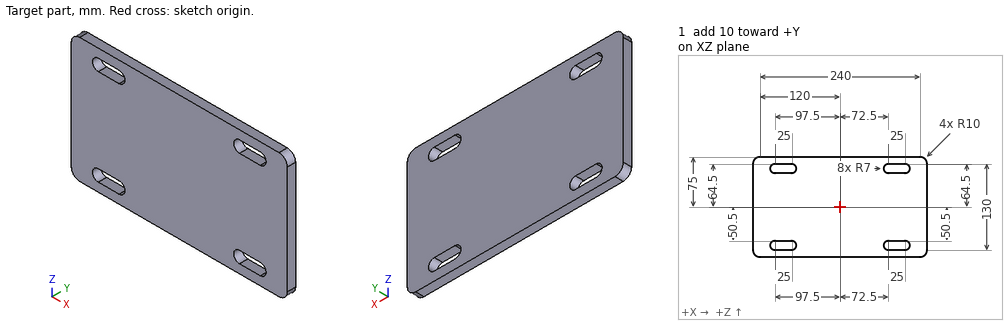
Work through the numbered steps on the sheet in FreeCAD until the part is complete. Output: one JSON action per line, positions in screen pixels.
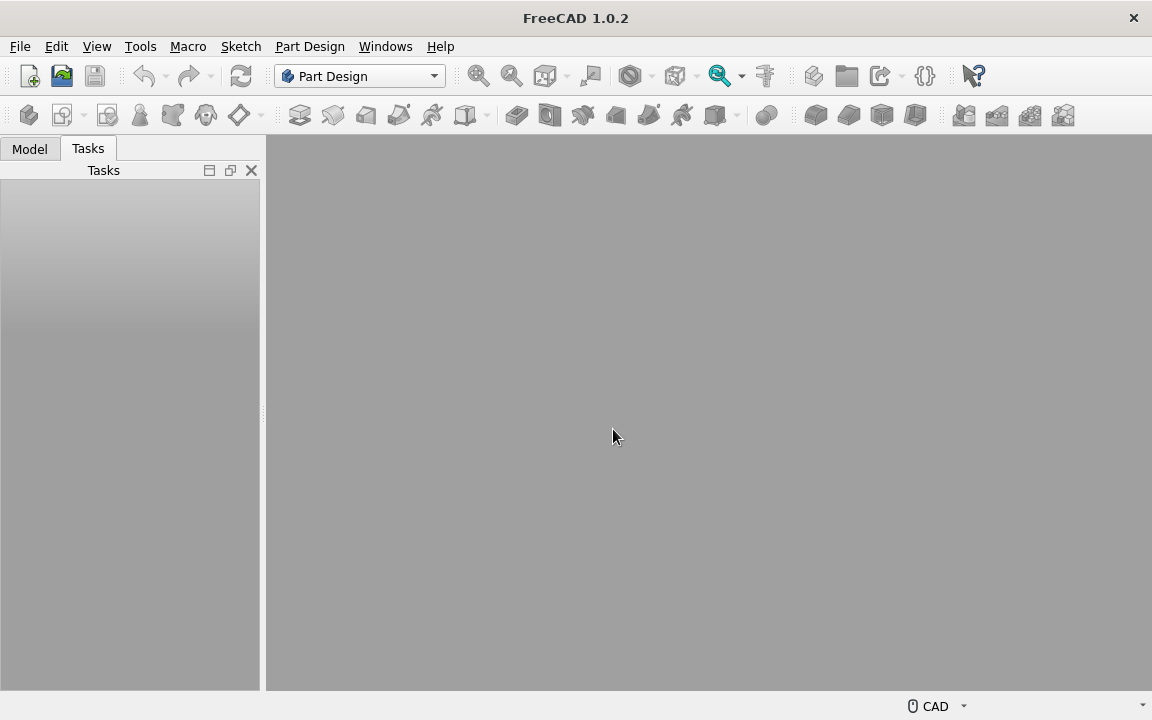
{"action": "left_click", "coordinate": [29, 76]}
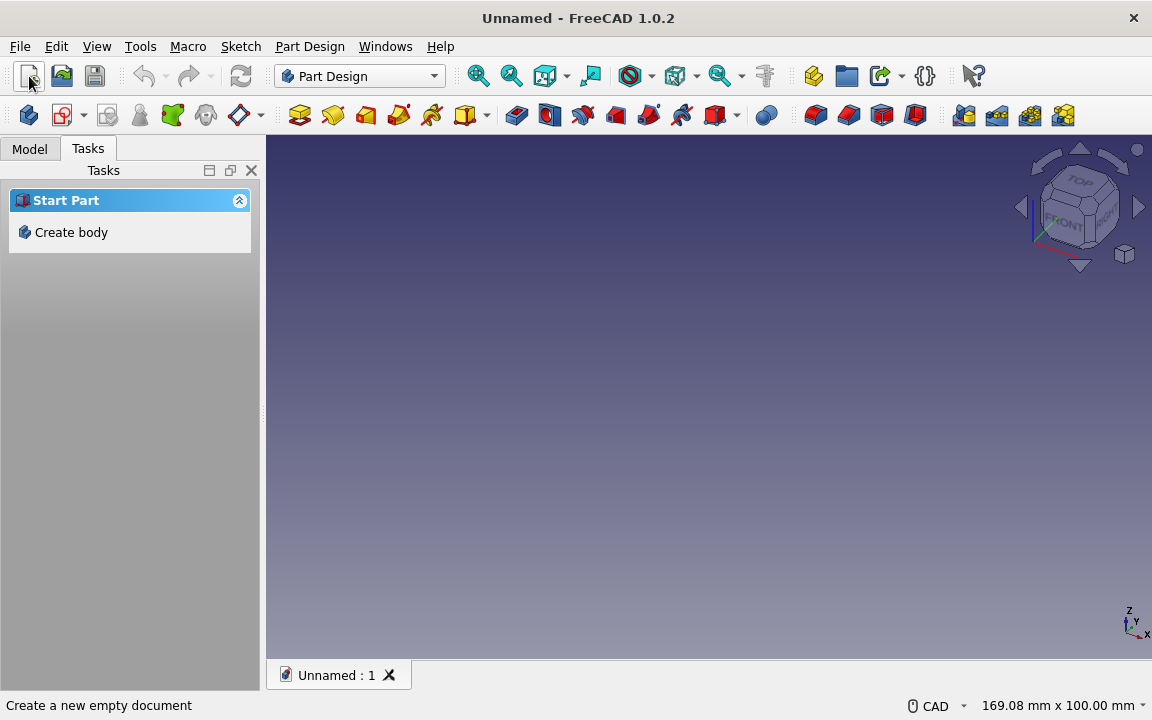
{"action": "left_click", "coordinate": [62, 116]}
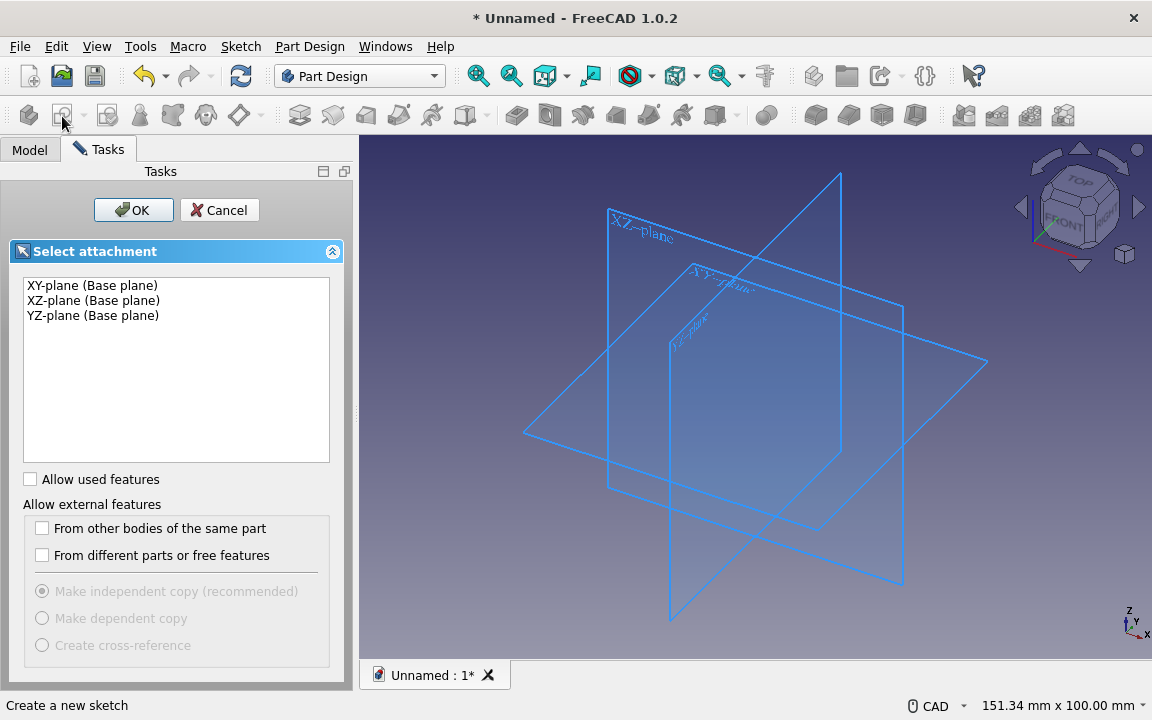
{"action": "left_click", "coordinate": [84, 300]}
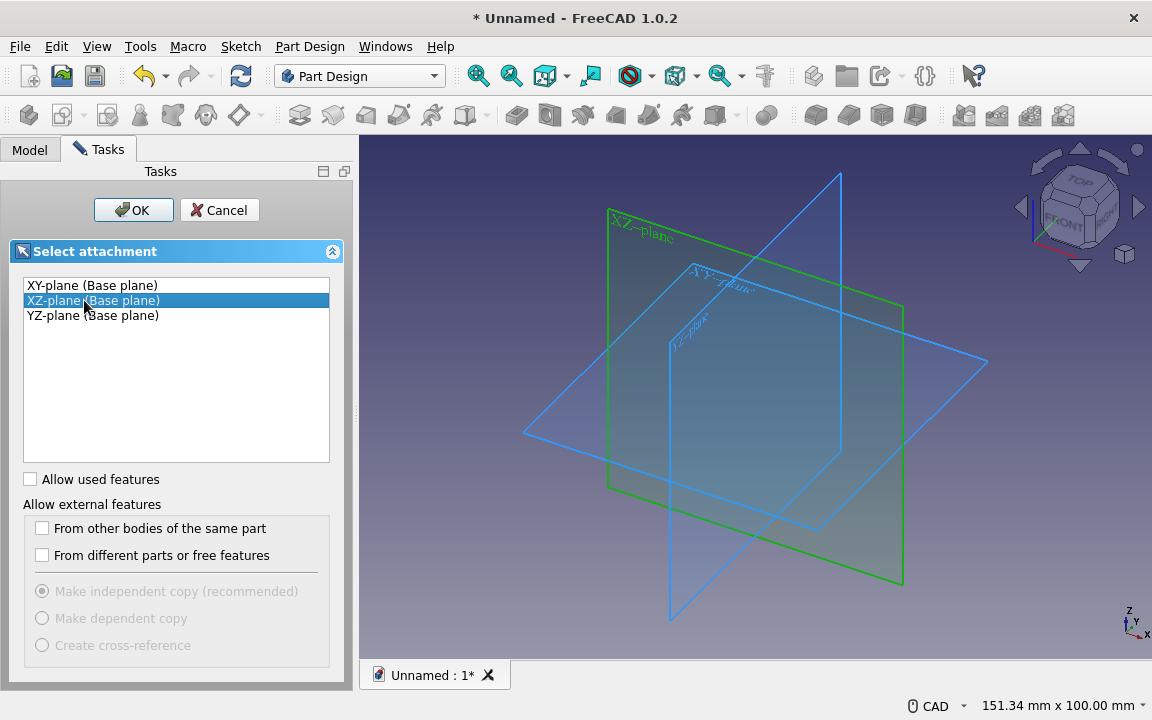
{"action": "left_click", "coordinate": [134, 210]}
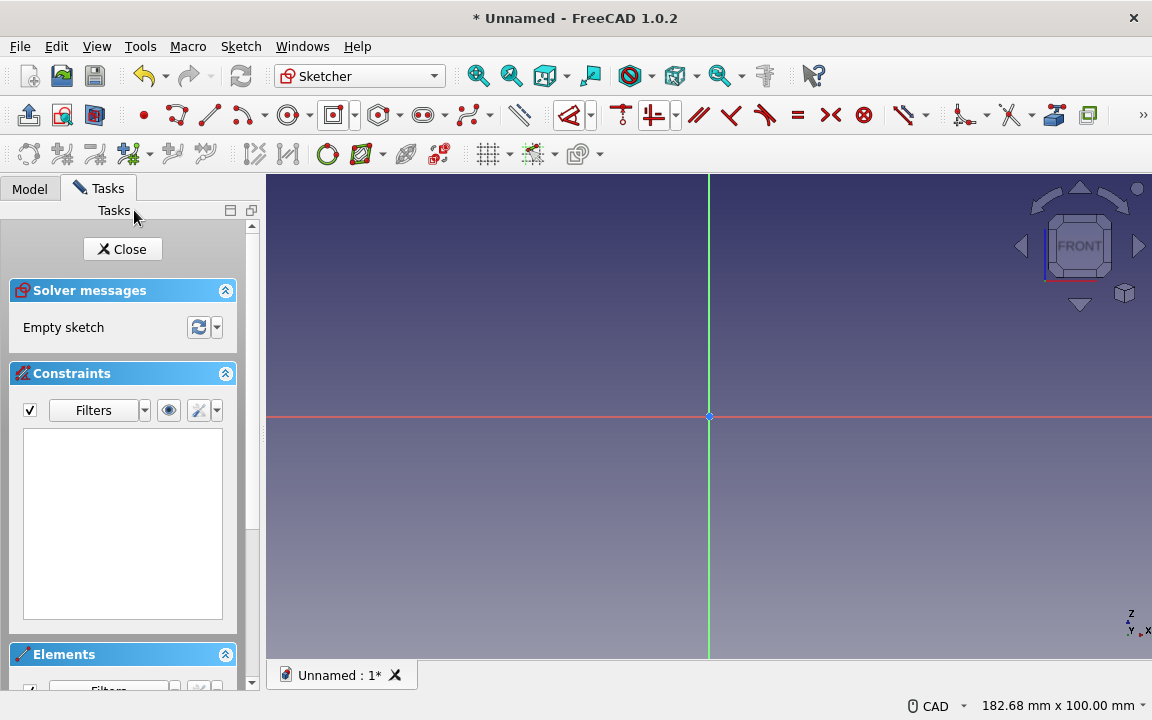
{"action": "scroll", "coordinate": [601, 417], "scroll_direction": "down", "scroll_amount": 5}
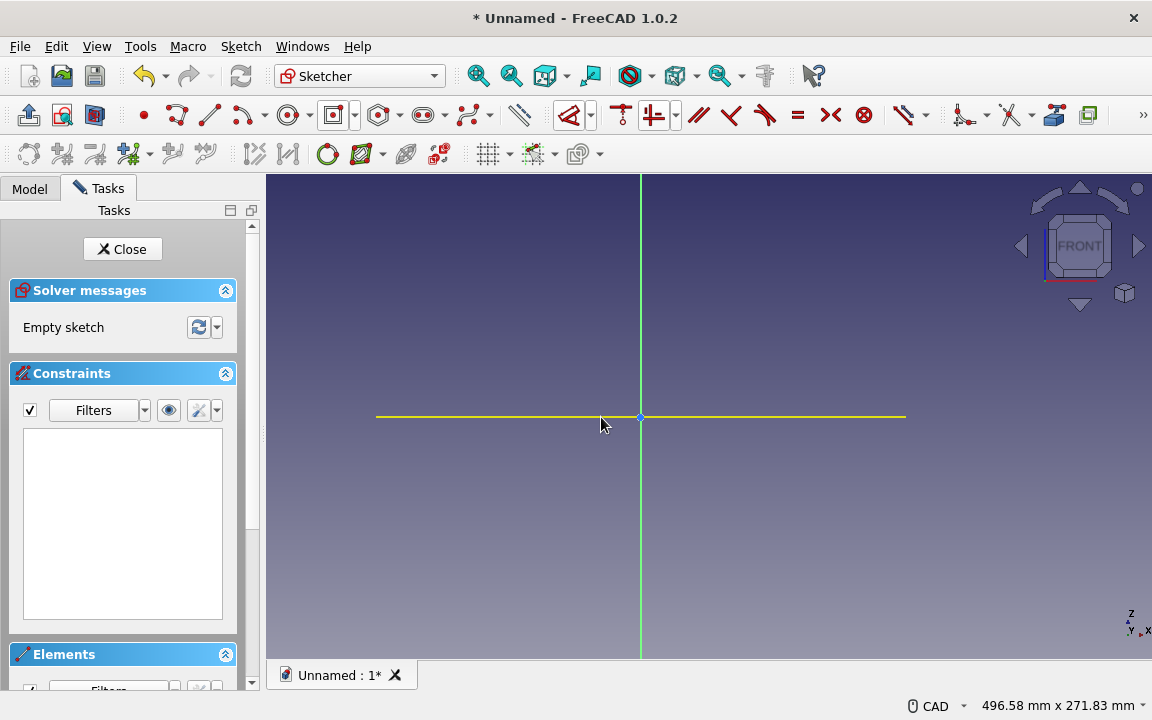
{"action": "left_click", "coordinate": [210, 116]}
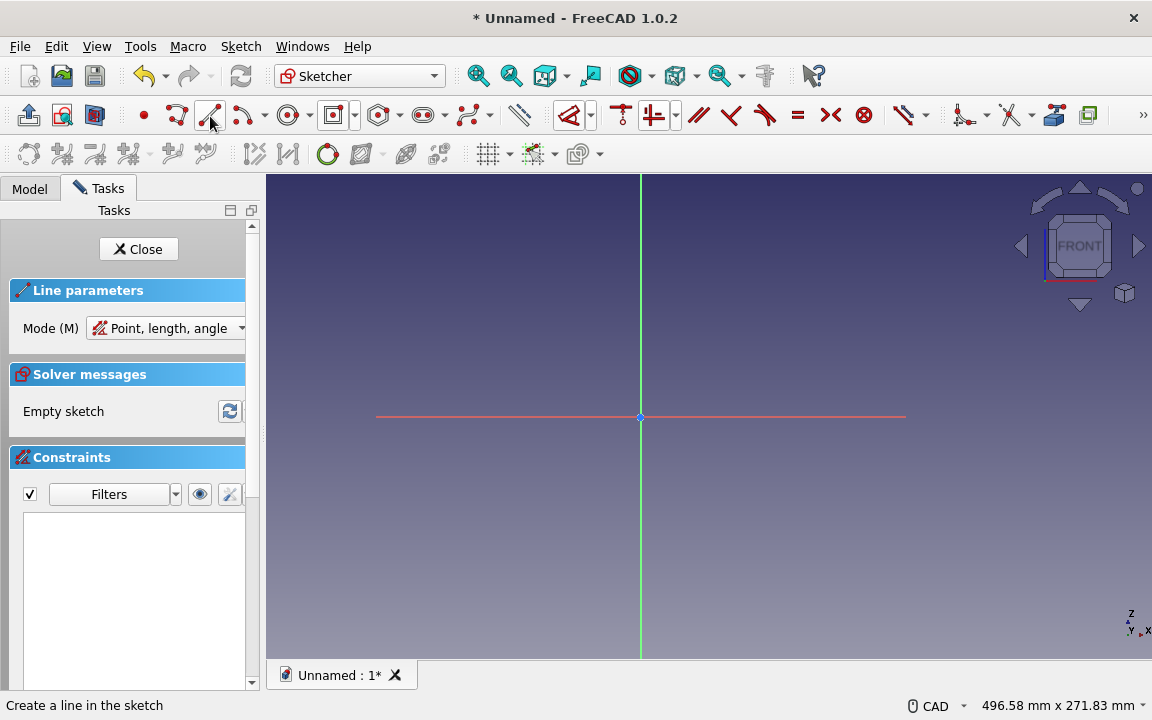
{"action": "left_click", "coordinate": [427, 283]}
{"action": "left_click", "coordinate": [855, 283]}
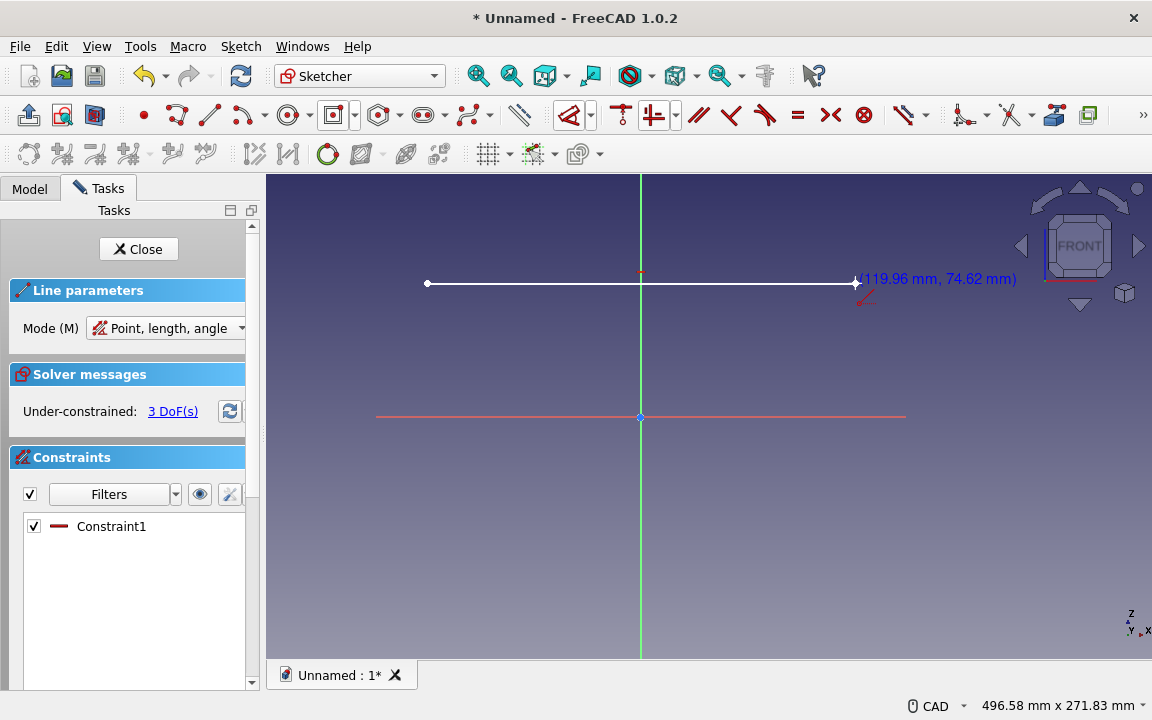
{"action": "left_click", "coordinate": [873, 301]}
{"action": "left_click", "coordinate": [873, 533]}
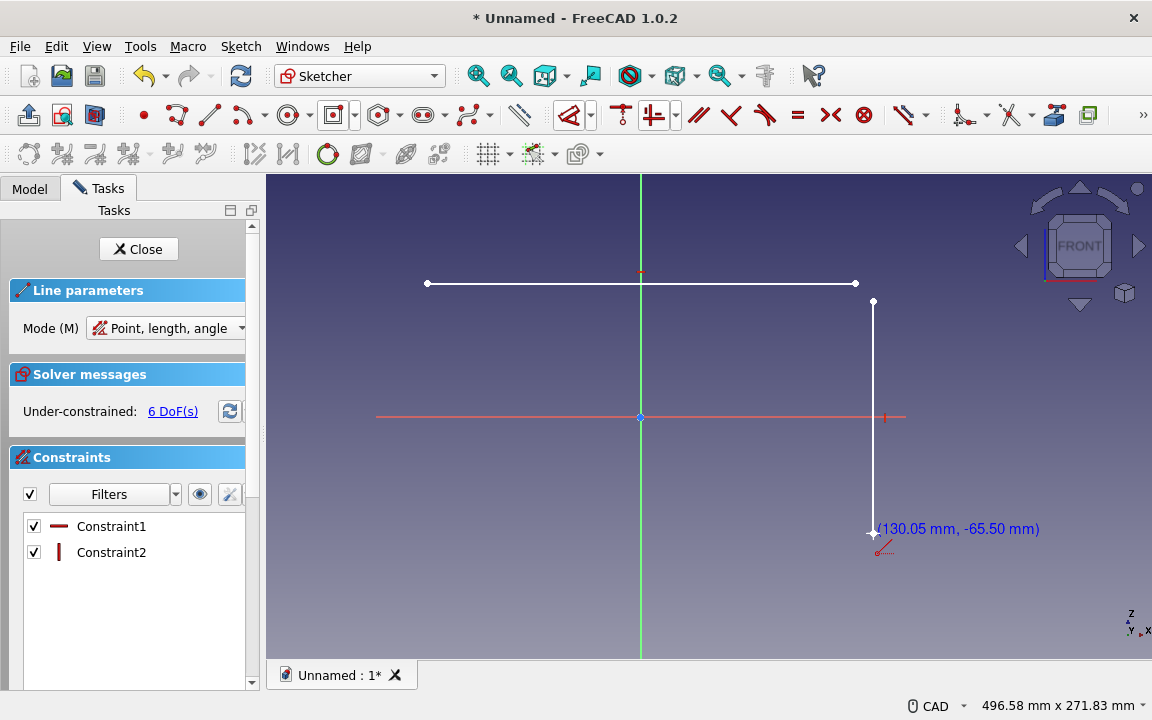
{"action": "left_click", "coordinate": [855, 551]}
{"action": "left_click", "coordinate": [427, 551]}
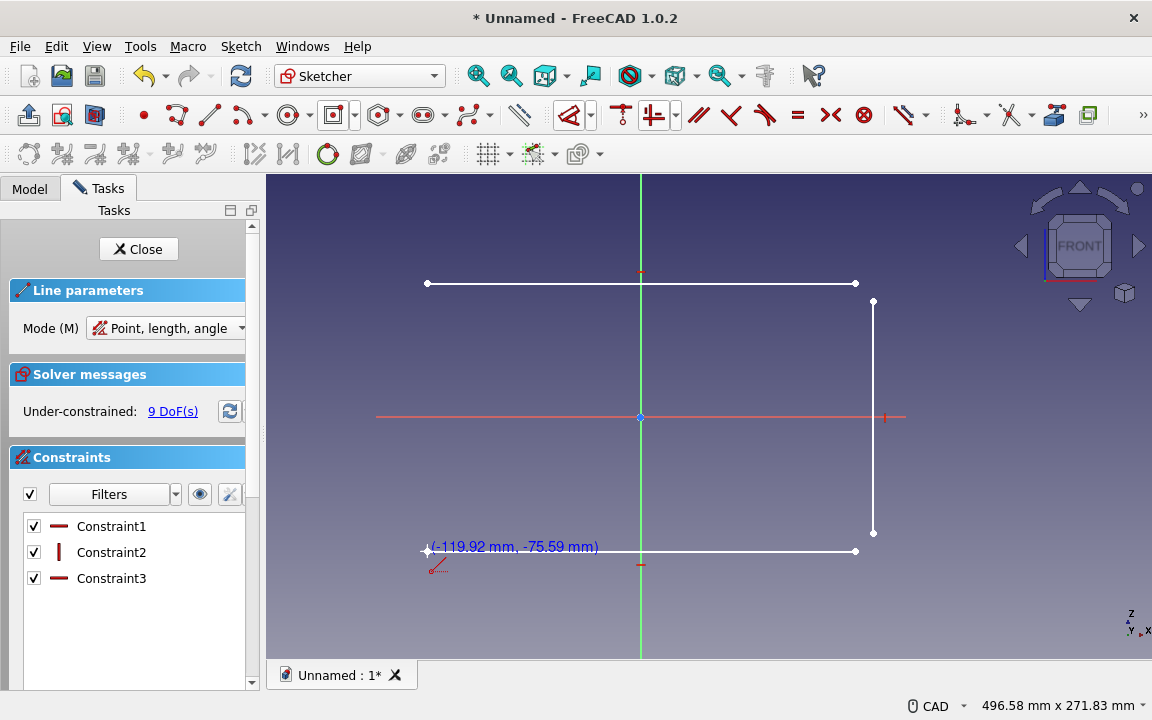
{"action": "left_click", "coordinate": [409, 533]}
{"action": "left_click", "coordinate": [409, 301]}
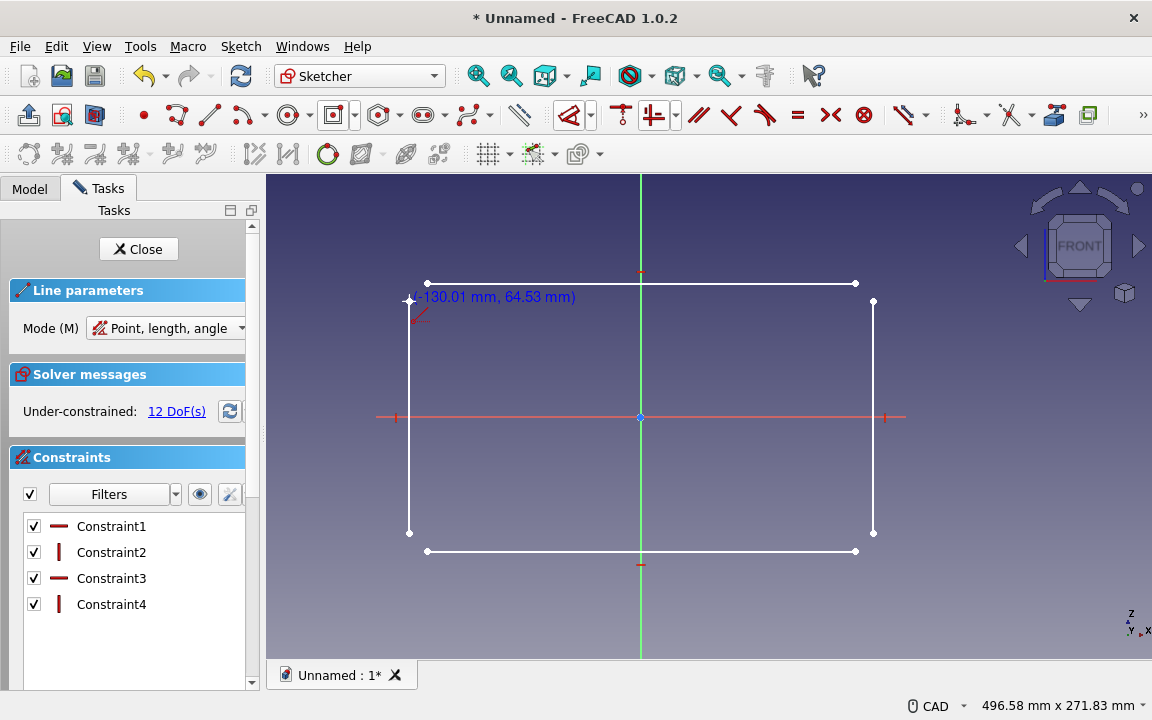
{"action": "left_click", "coordinate": [264, 116]}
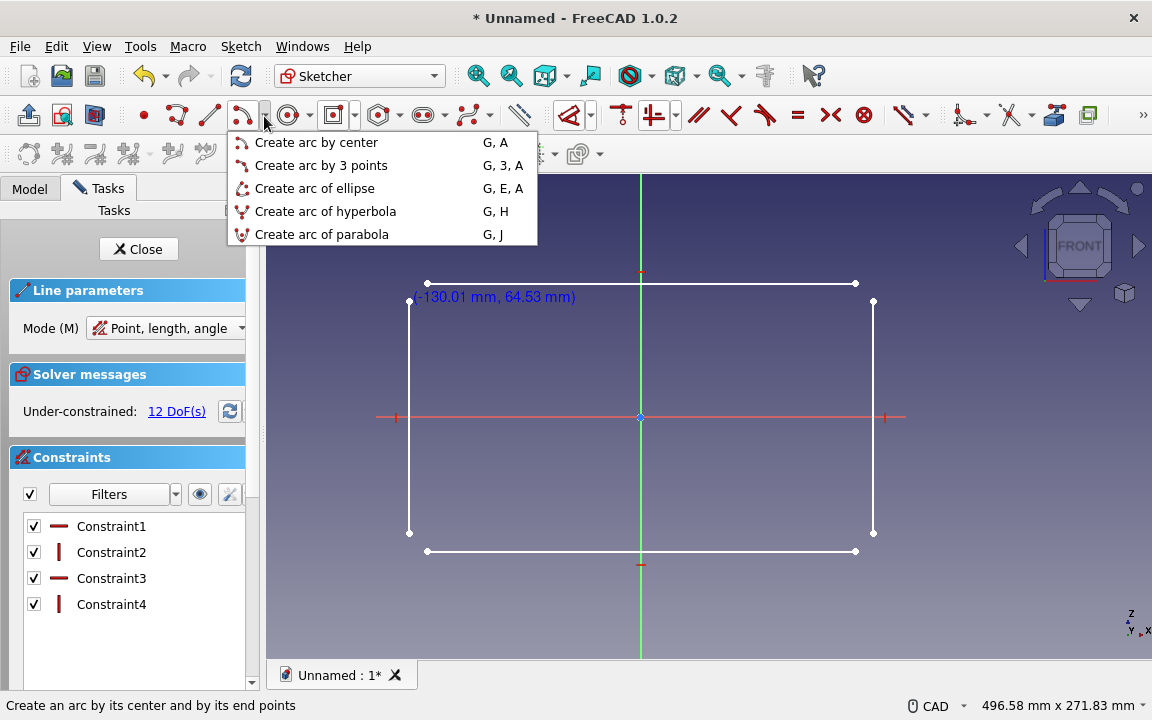
{"action": "left_click", "coordinate": [382, 166]}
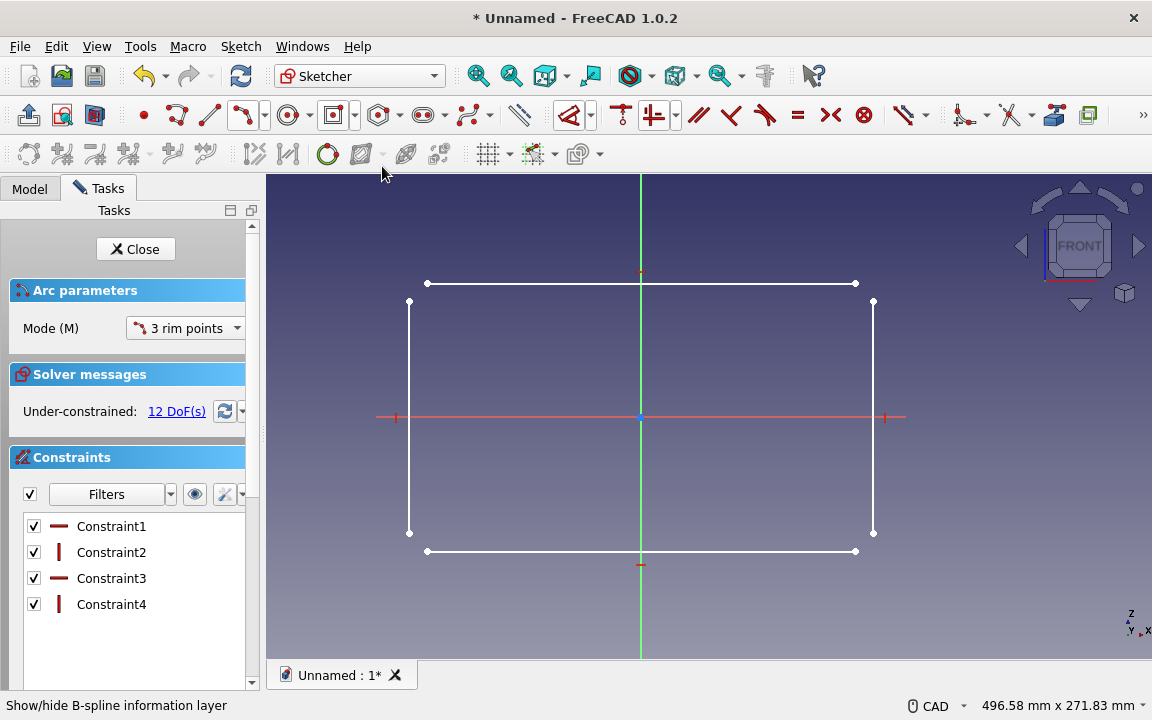
{"action": "left_click", "coordinate": [855, 284]}
{"action": "left_click", "coordinate": [873, 302]}